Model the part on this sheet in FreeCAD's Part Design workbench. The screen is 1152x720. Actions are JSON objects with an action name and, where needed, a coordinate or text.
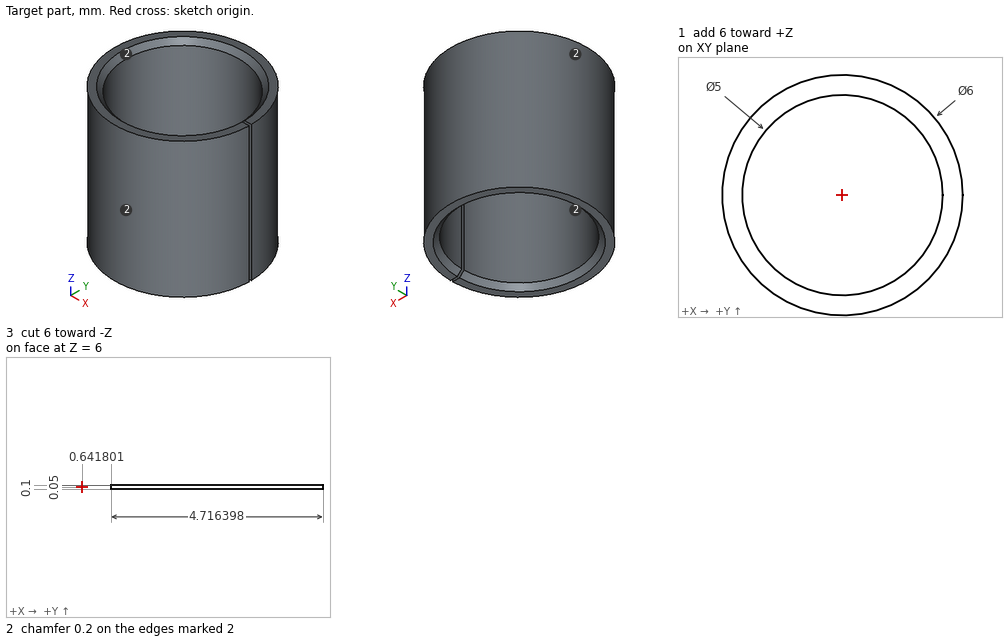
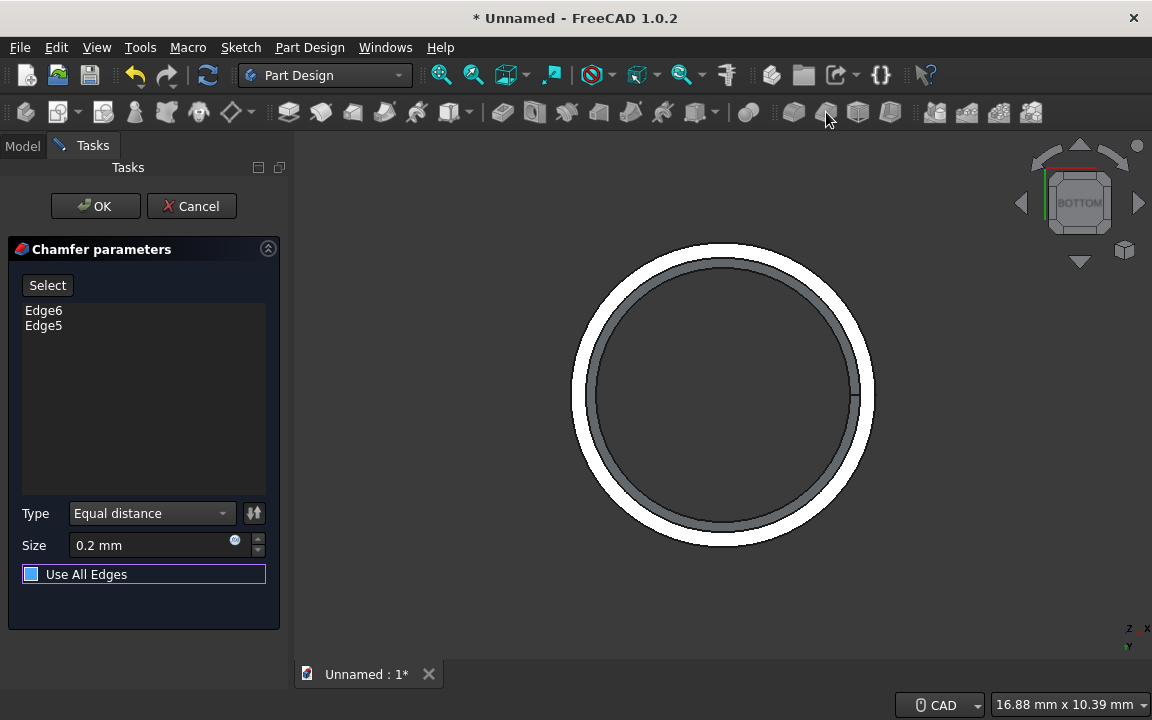
{"action": "left_click", "coordinate": [96, 206]}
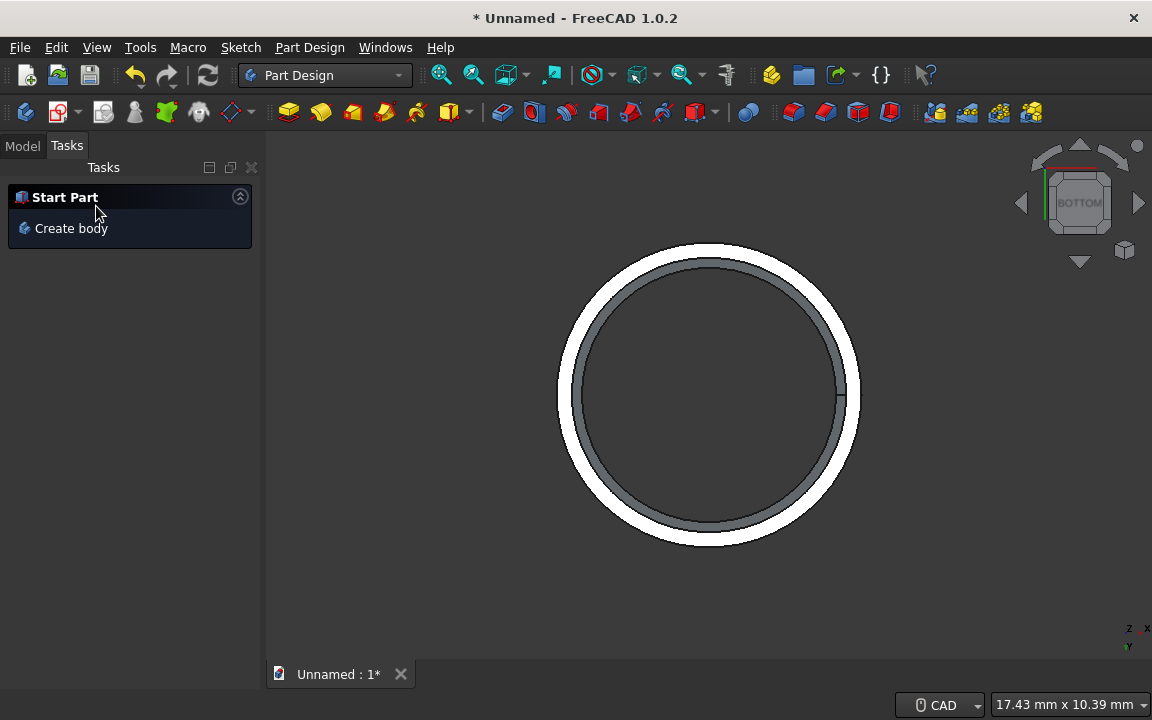
{"action": "key", "text": "0"}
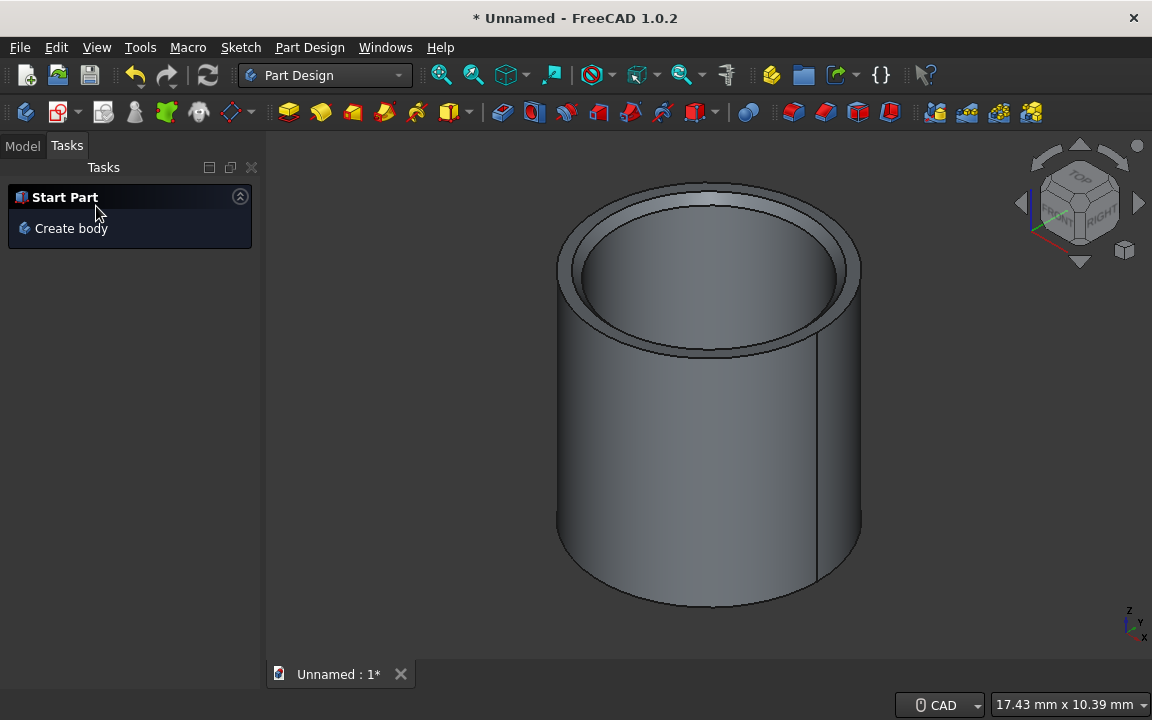
{"action": "scroll", "coordinate": [647, 198], "scroll_direction": "up", "scroll_amount": 15}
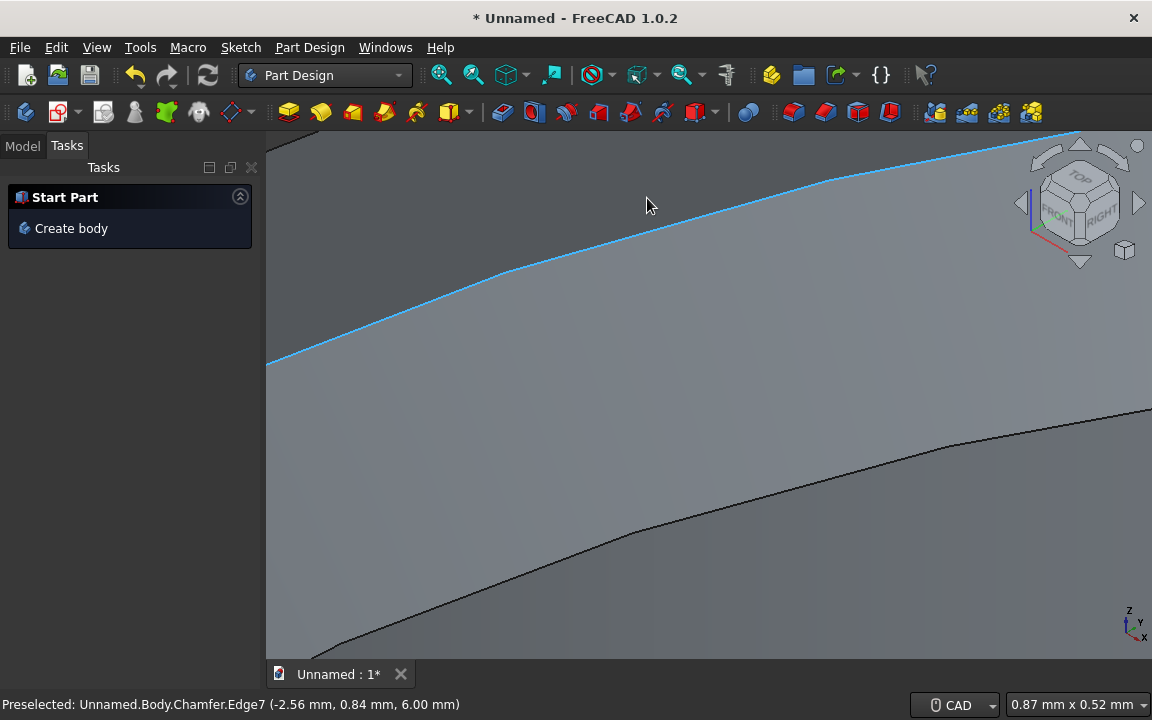
{"action": "left_click", "coordinate": [646, 221]}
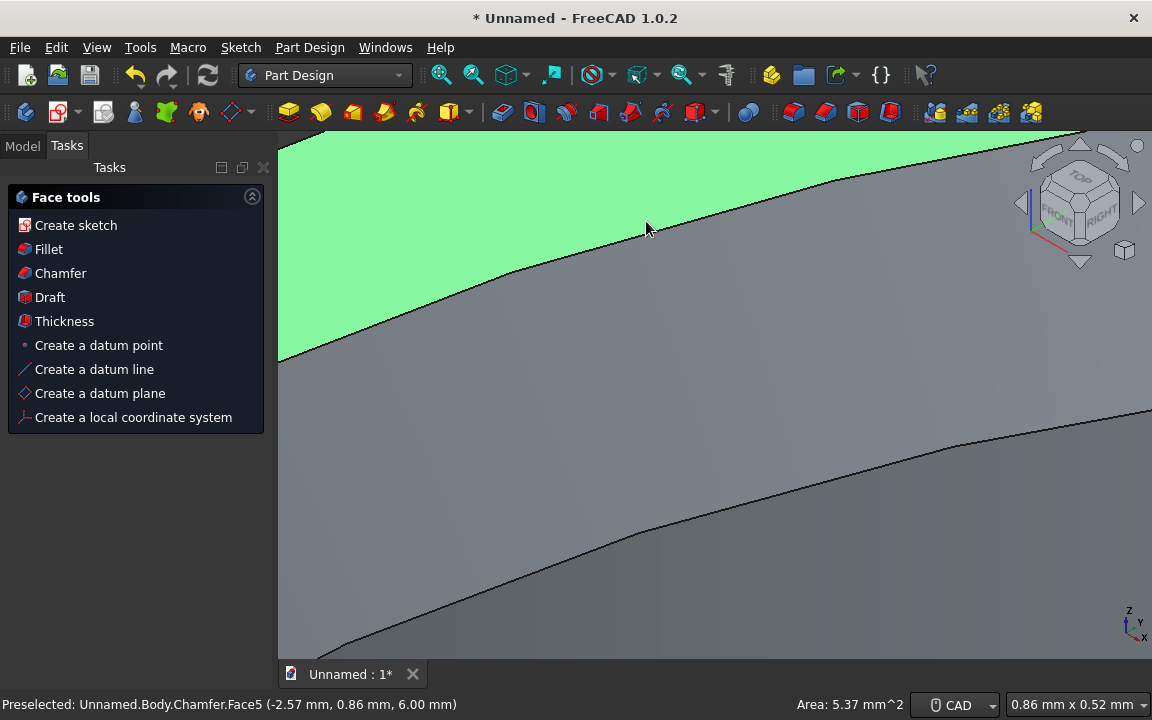
{"action": "left_click", "coordinate": [58, 112]}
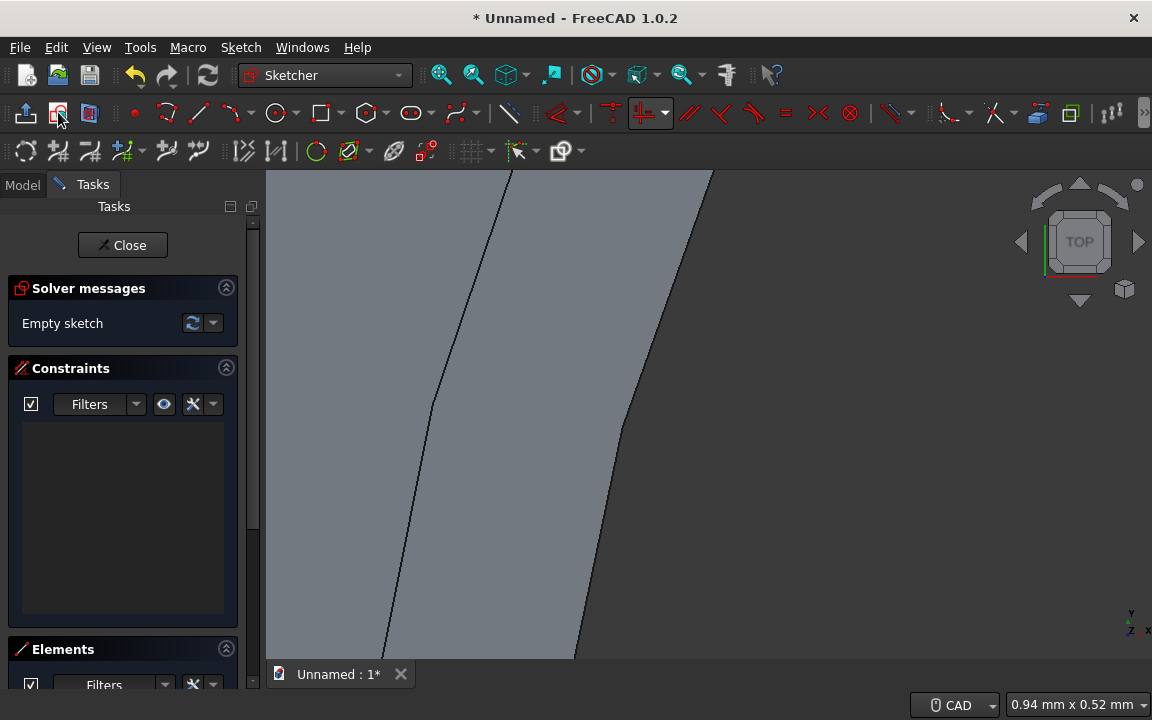
{"action": "scroll", "coordinate": [294, 362], "scroll_direction": "down", "scroll_amount": 13}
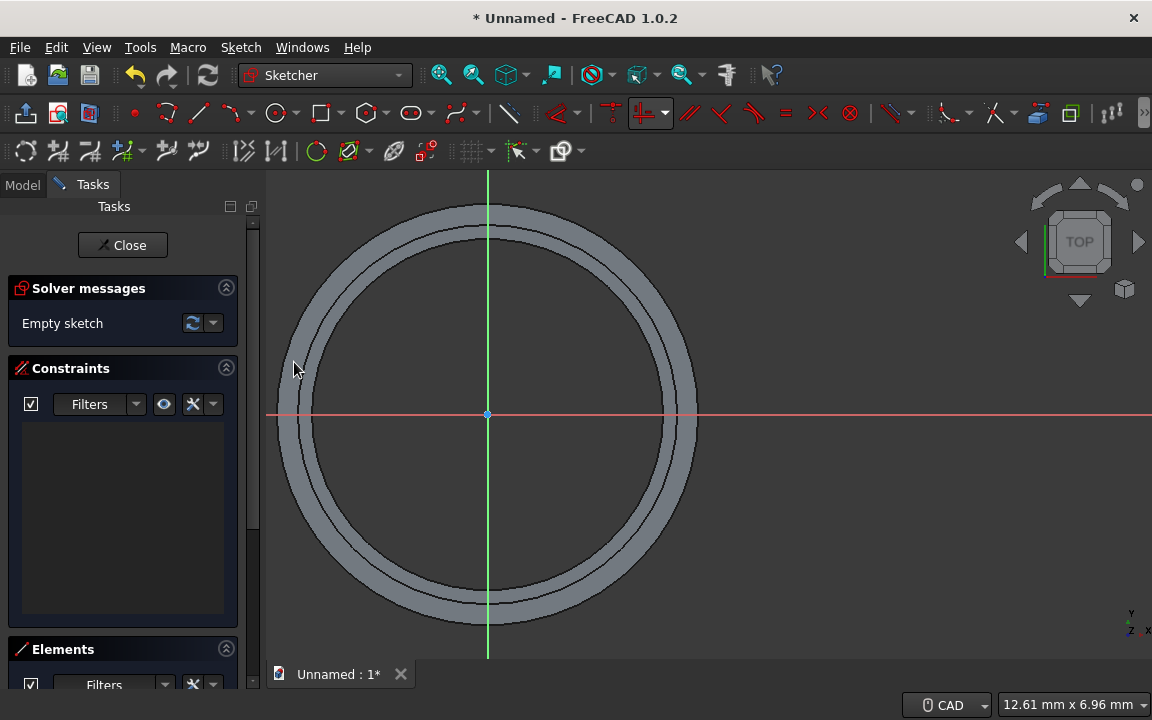
{"action": "left_click", "coordinate": [322, 114]}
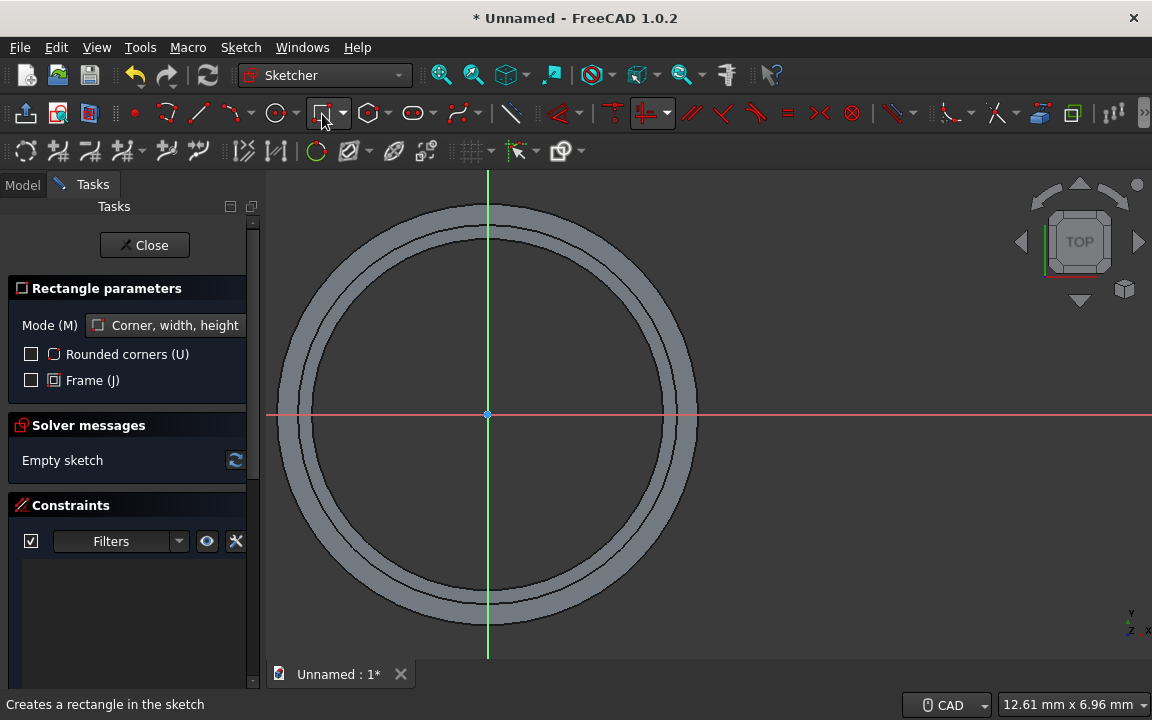
{"action": "scroll", "coordinate": [533, 411], "scroll_direction": "up", "scroll_amount": 8}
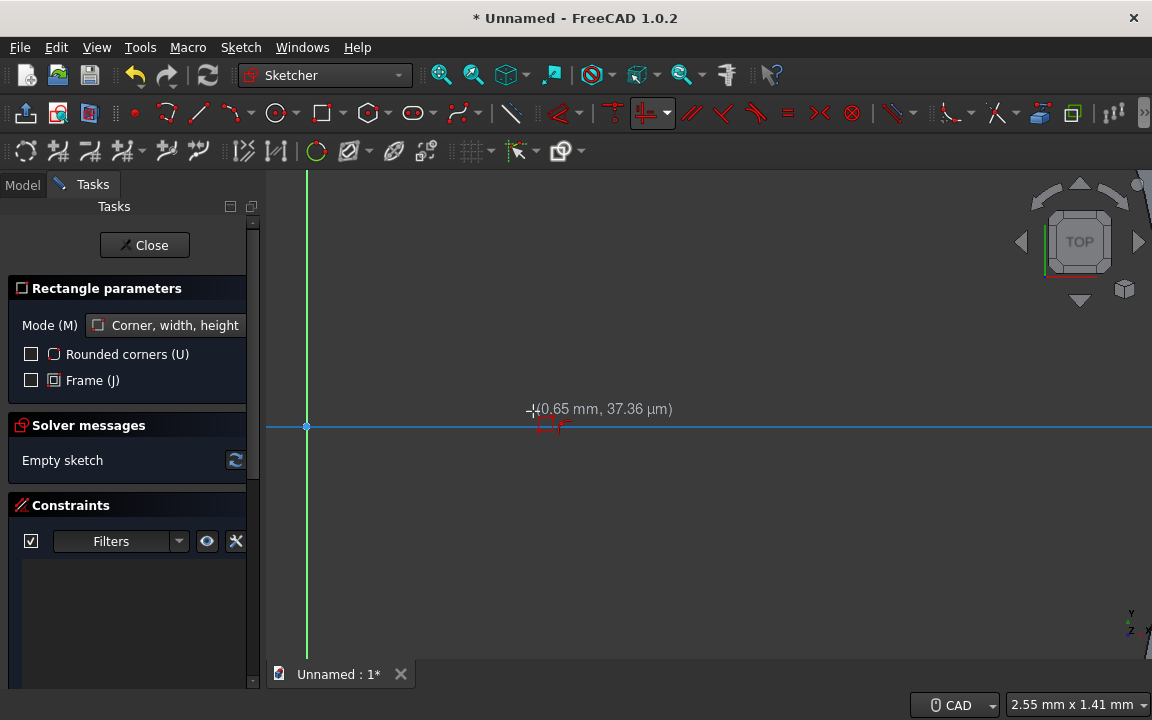
{"action": "left_click", "coordinate": [530, 410]}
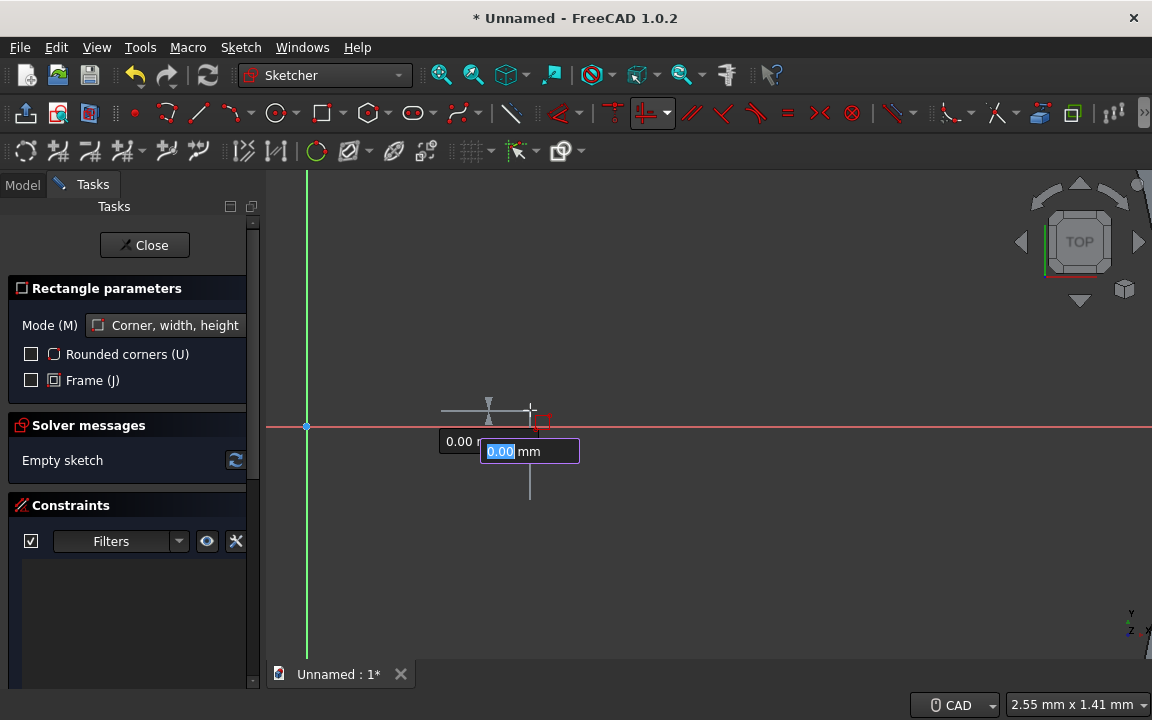
{"action": "scroll", "coordinate": [445, 410], "scroll_direction": "down", "scroll_amount": 7}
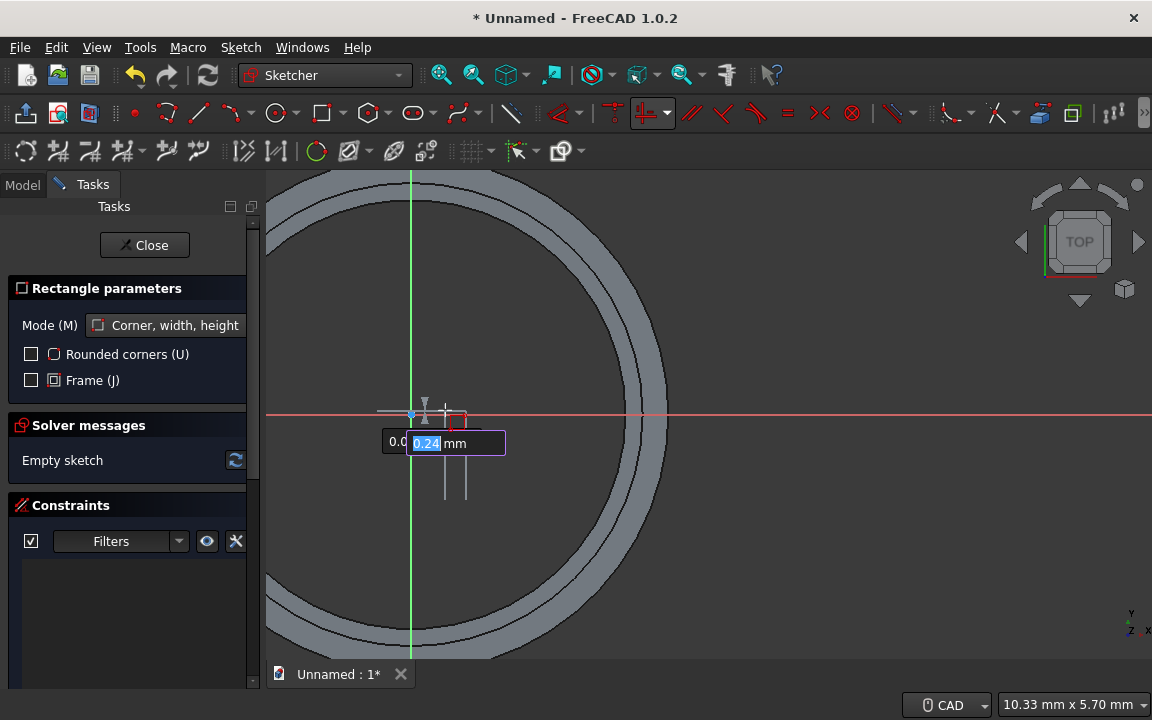
{"action": "scroll", "coordinate": [871, 419], "scroll_direction": "up", "scroll_amount": 7}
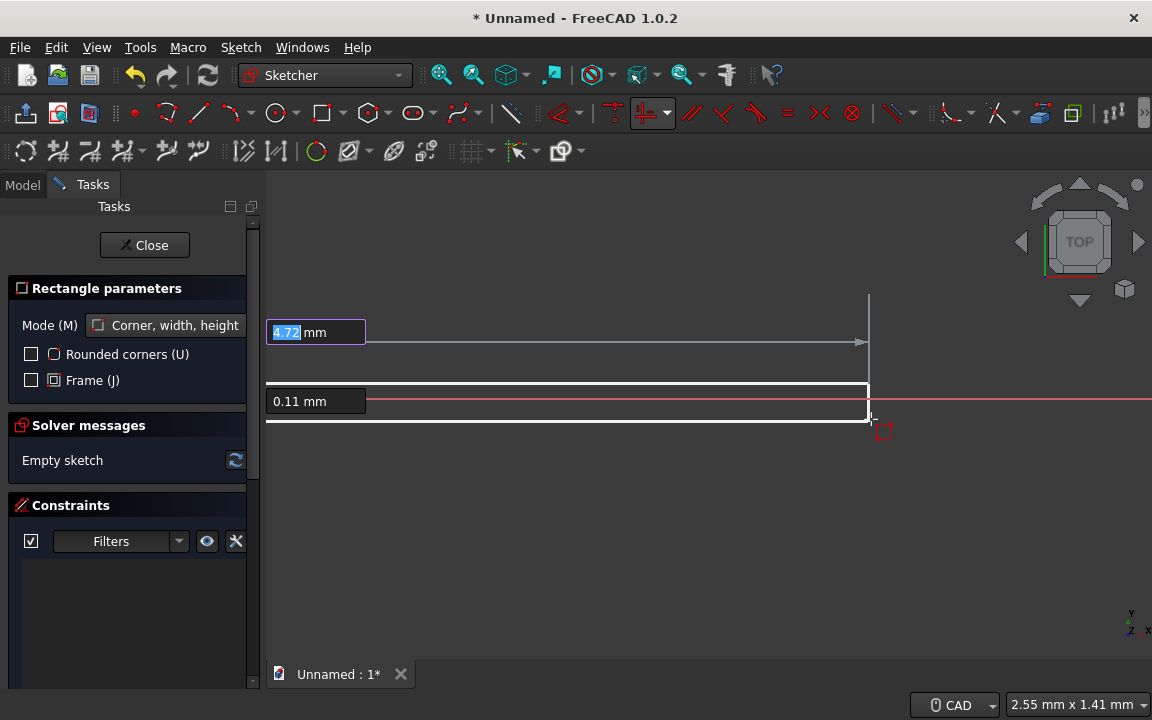
{"action": "left_click", "coordinate": [868, 417]}
{"action": "key", "text": "Escape"}